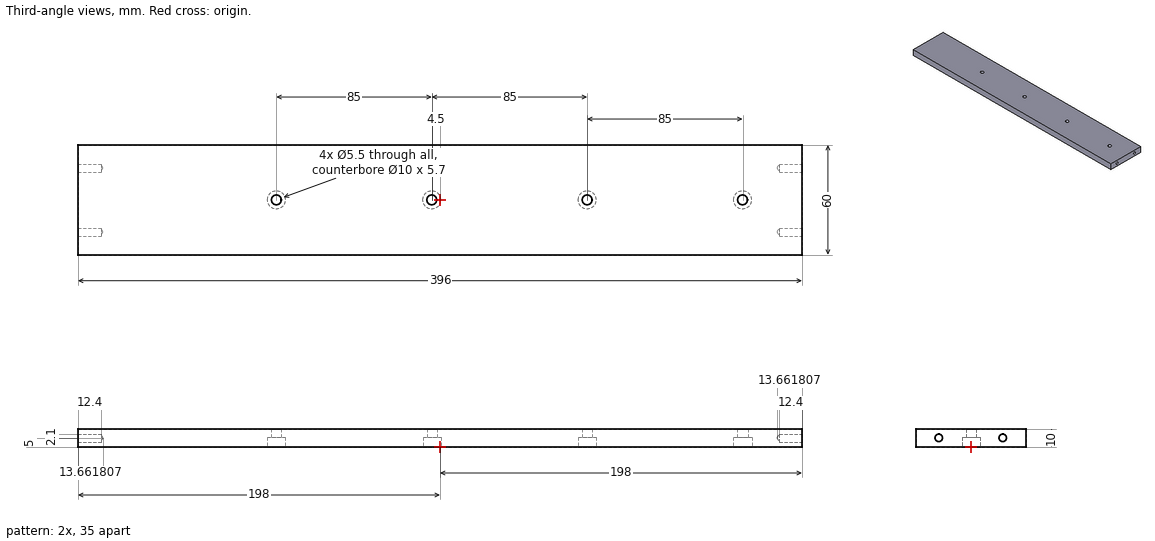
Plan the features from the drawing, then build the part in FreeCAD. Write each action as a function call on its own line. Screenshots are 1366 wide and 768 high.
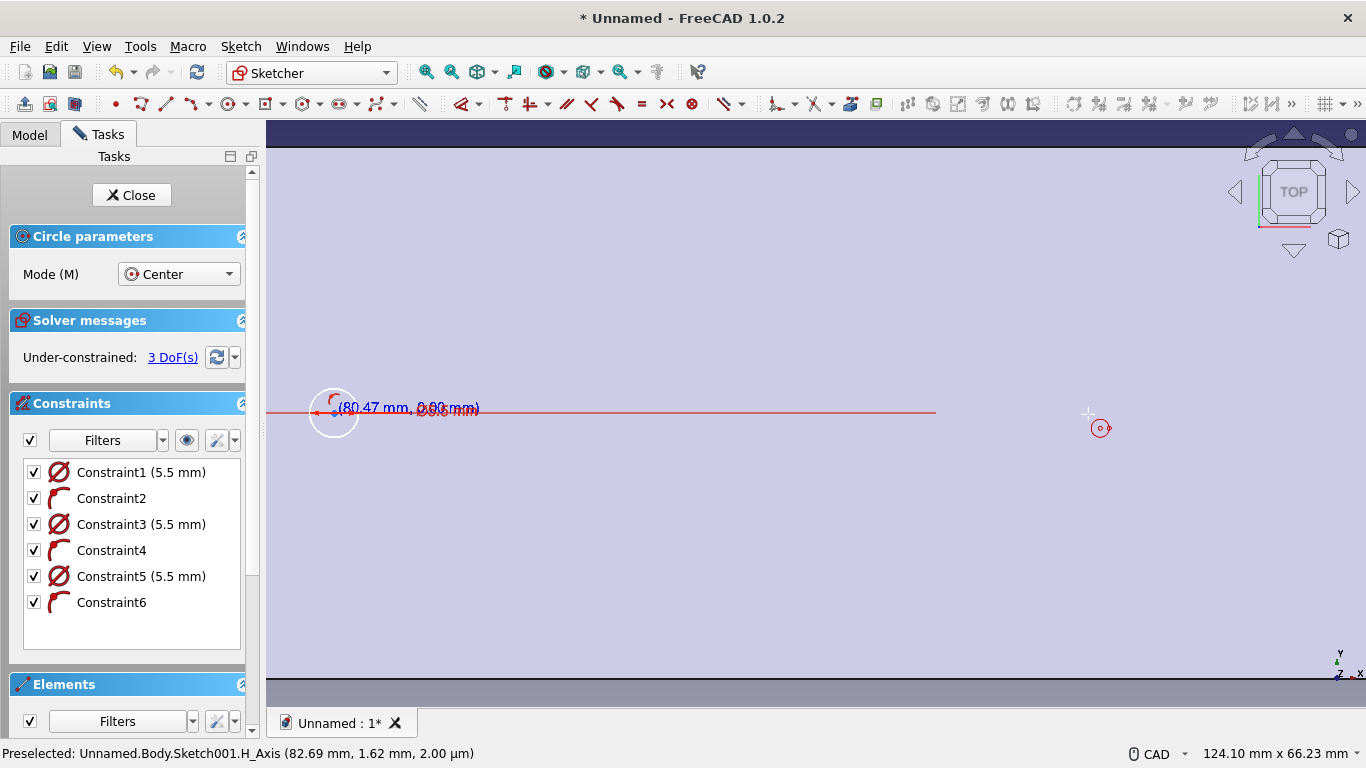
click(1088, 413)
move(1105, 396)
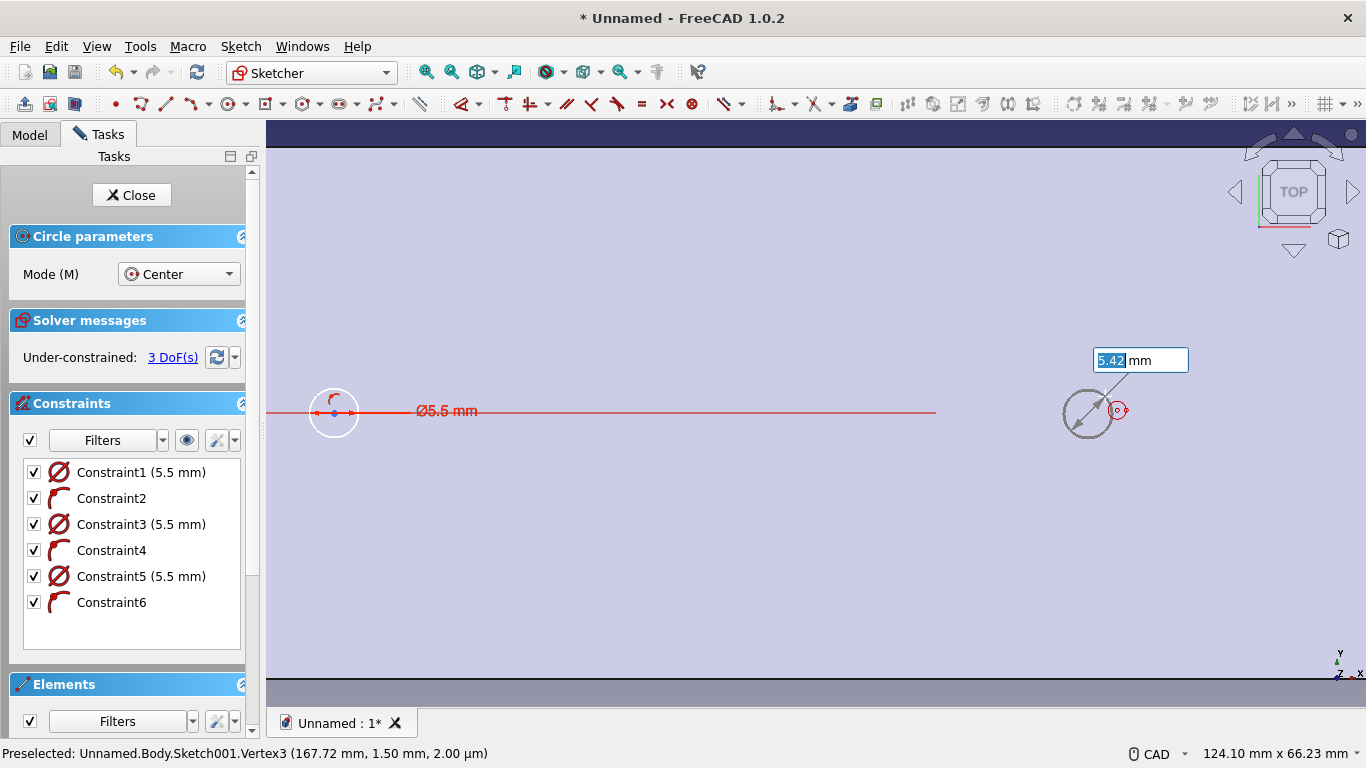
text(5.5)
key(Return)
key(Escape)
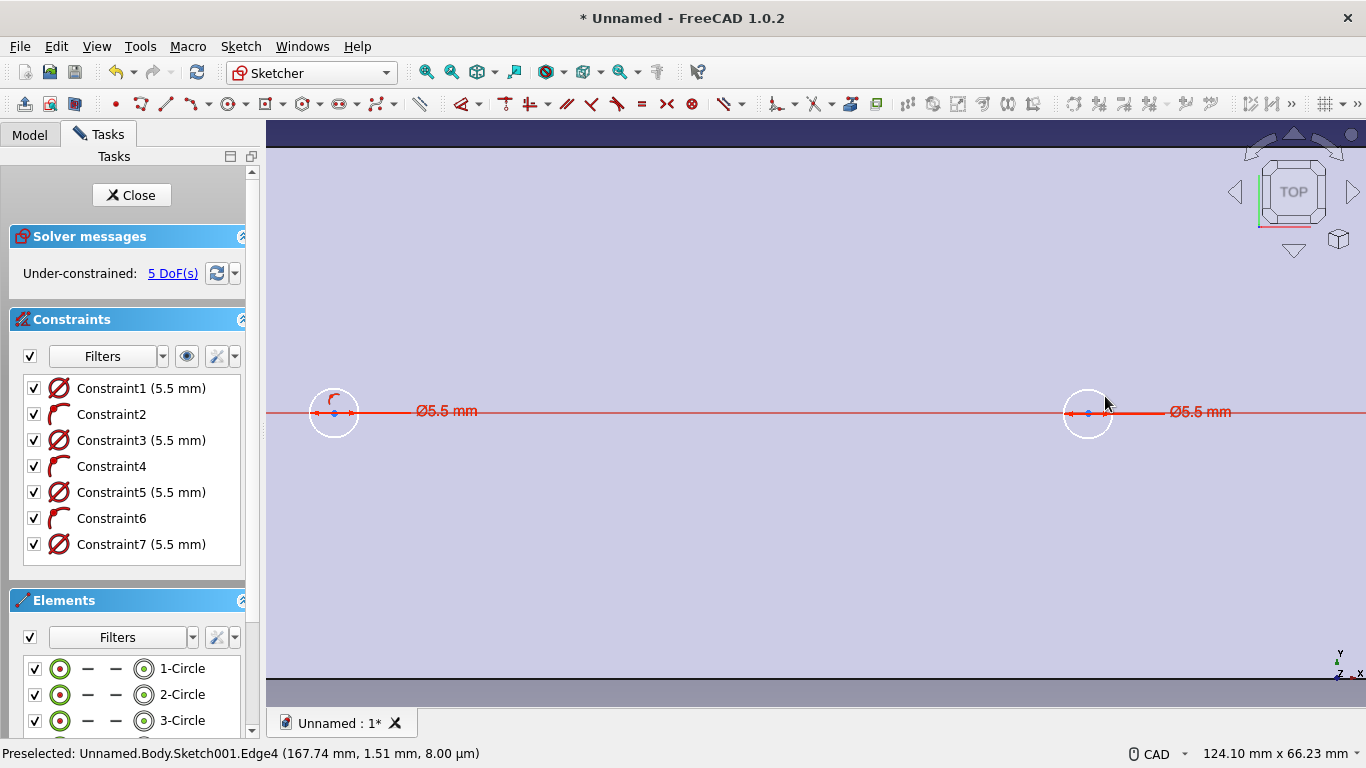
click(1088, 414)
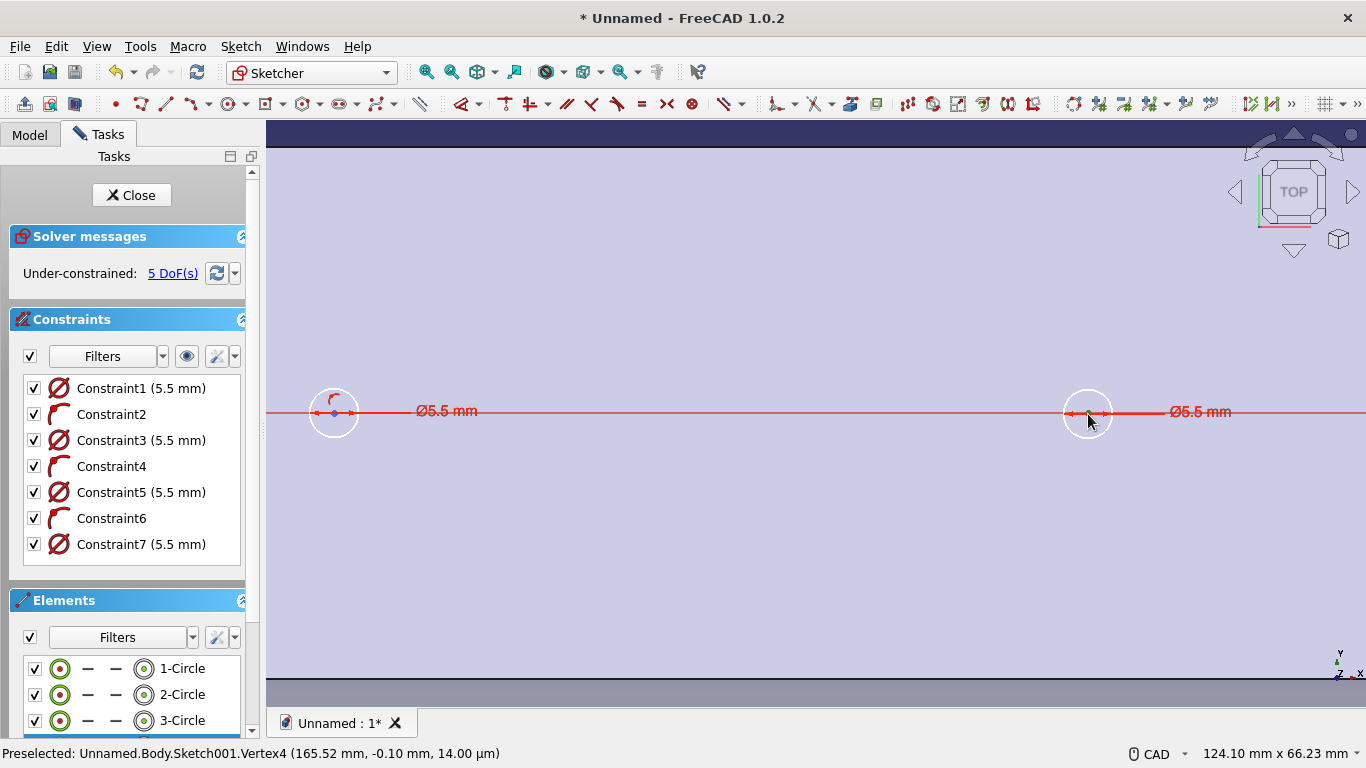
click(488, 413)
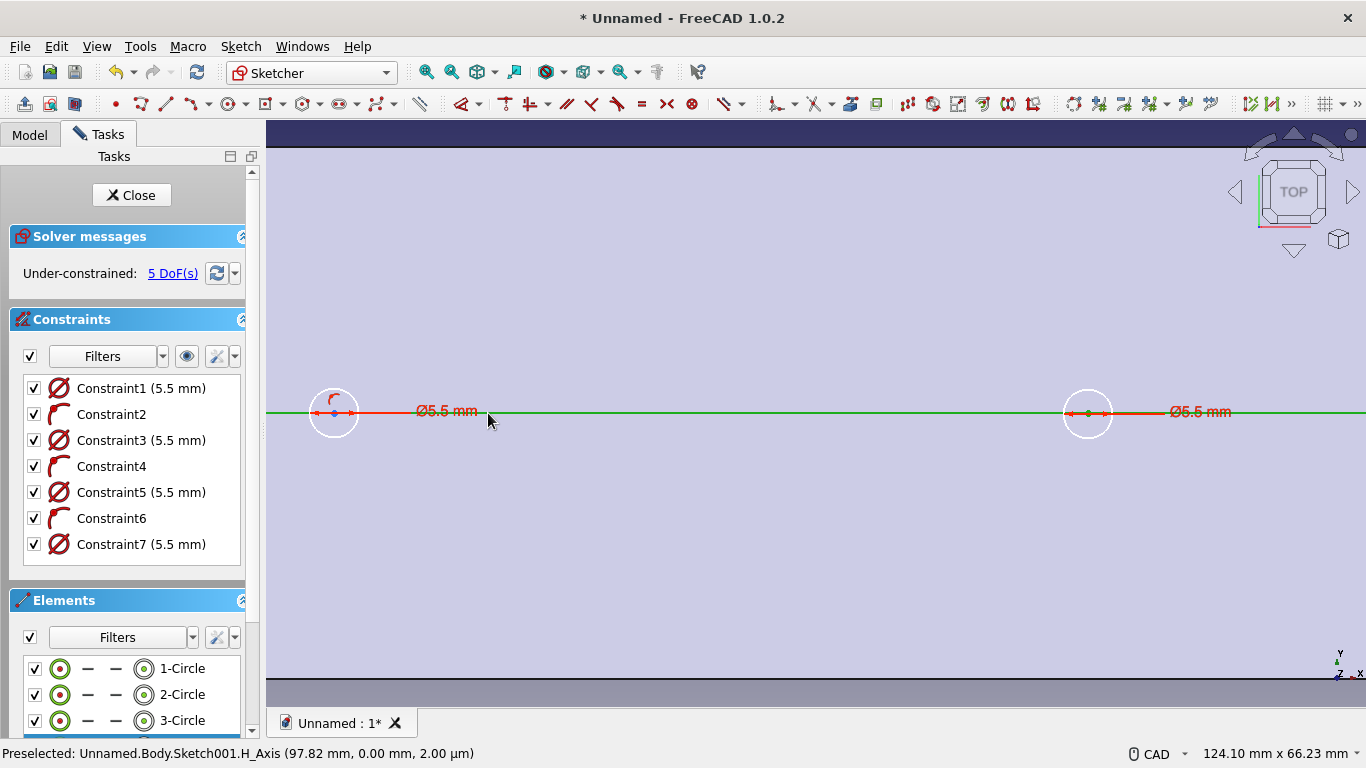
click(505, 104)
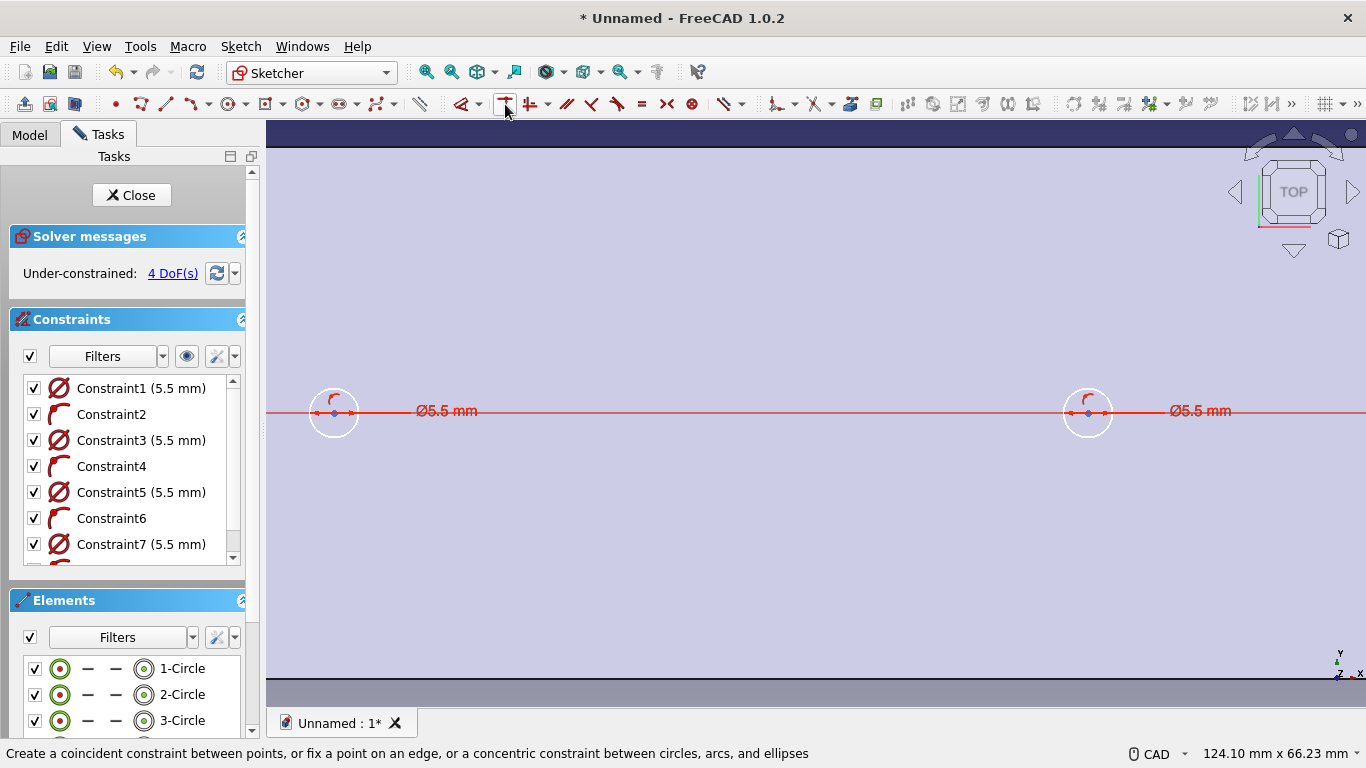
click(460, 104)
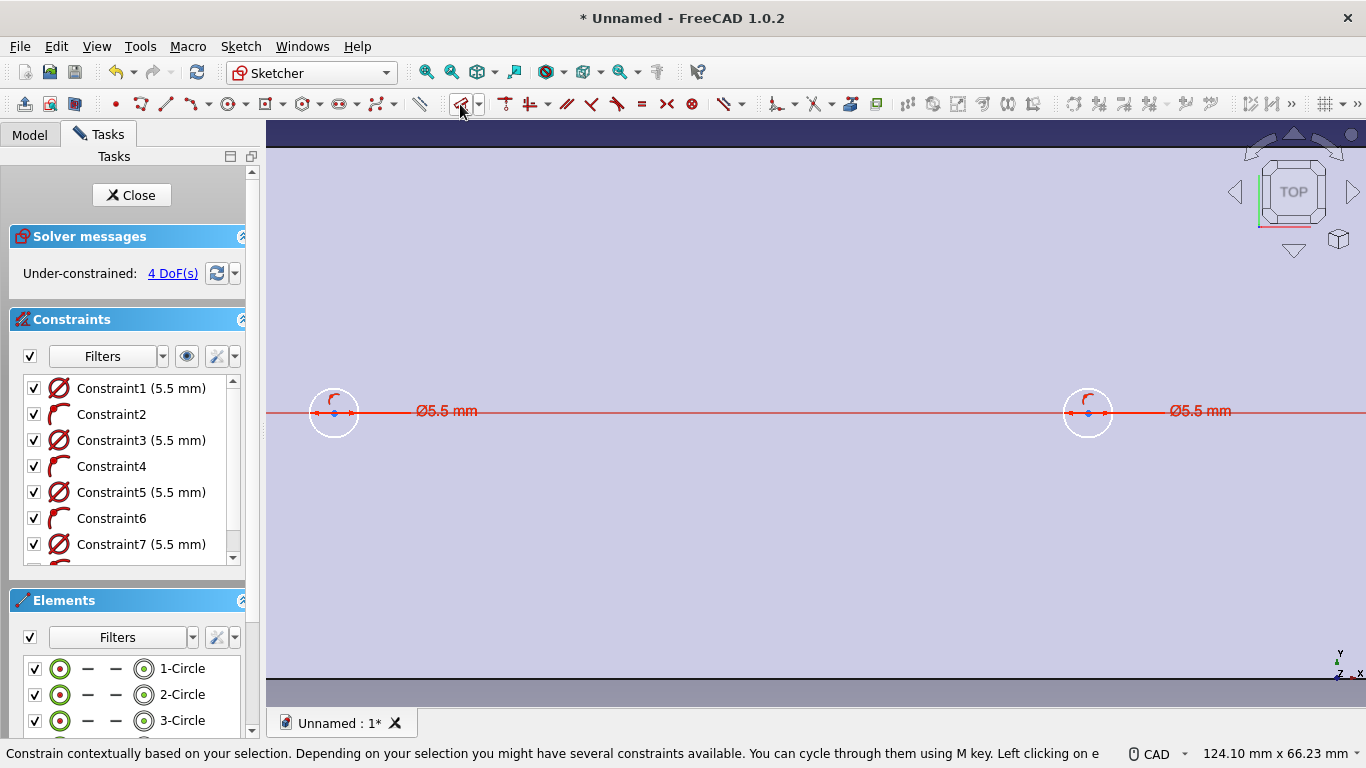
scroll(1088, 414, down, 6)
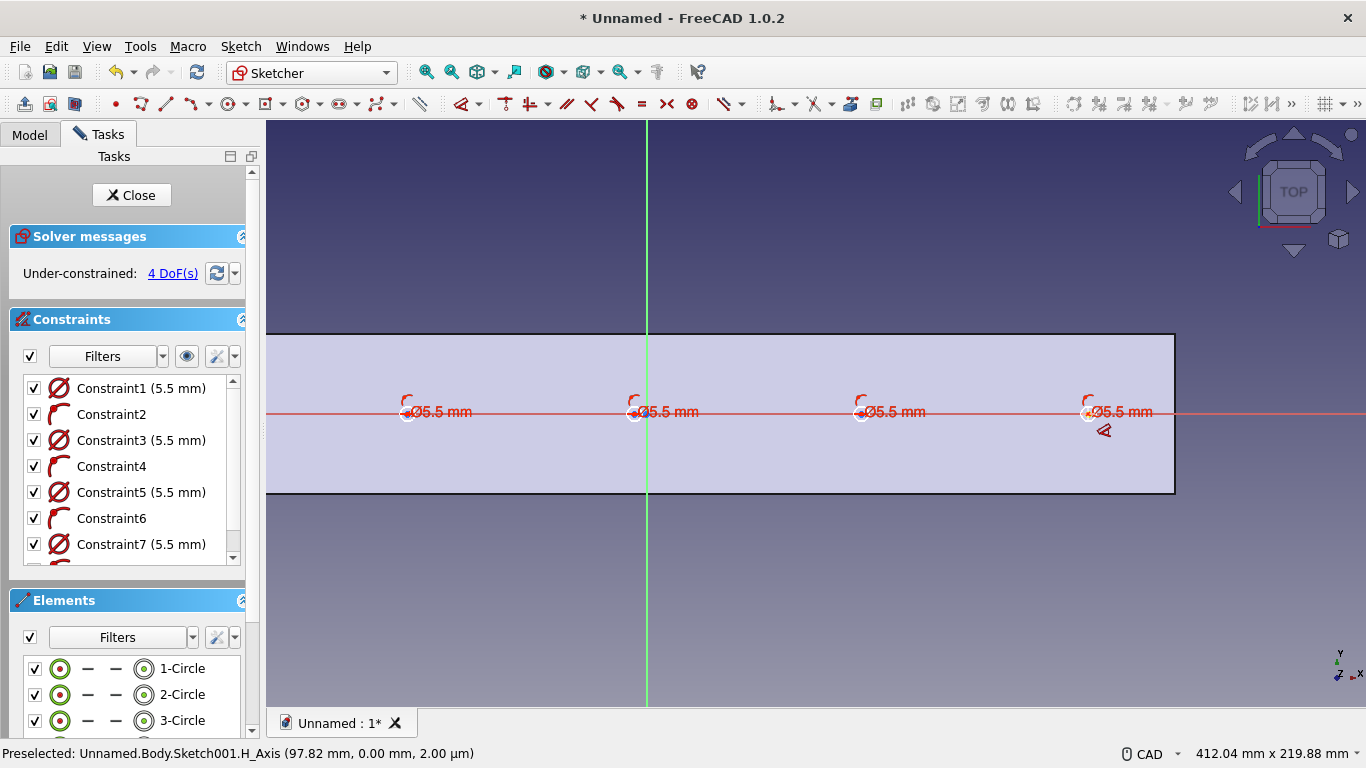
scroll(635, 414, up, 6)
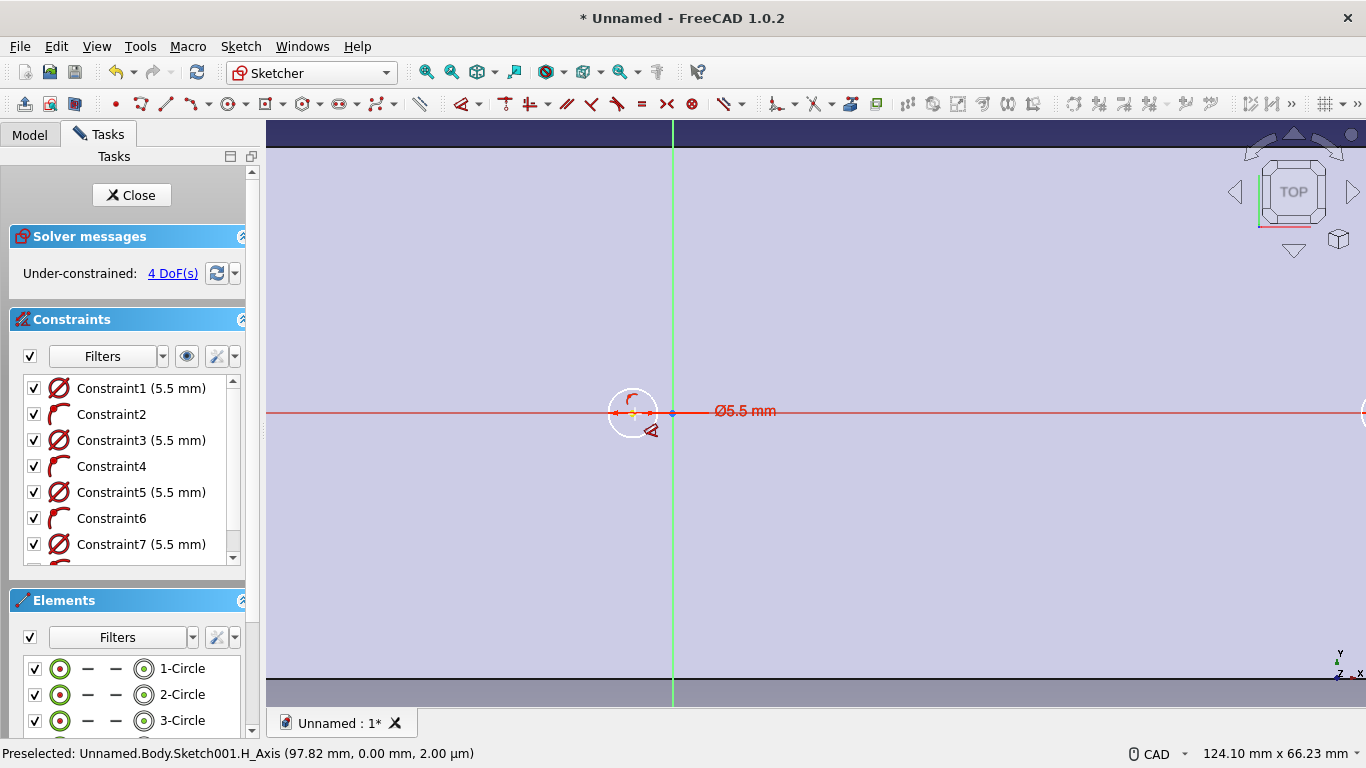
click(633, 413)
click(653, 447)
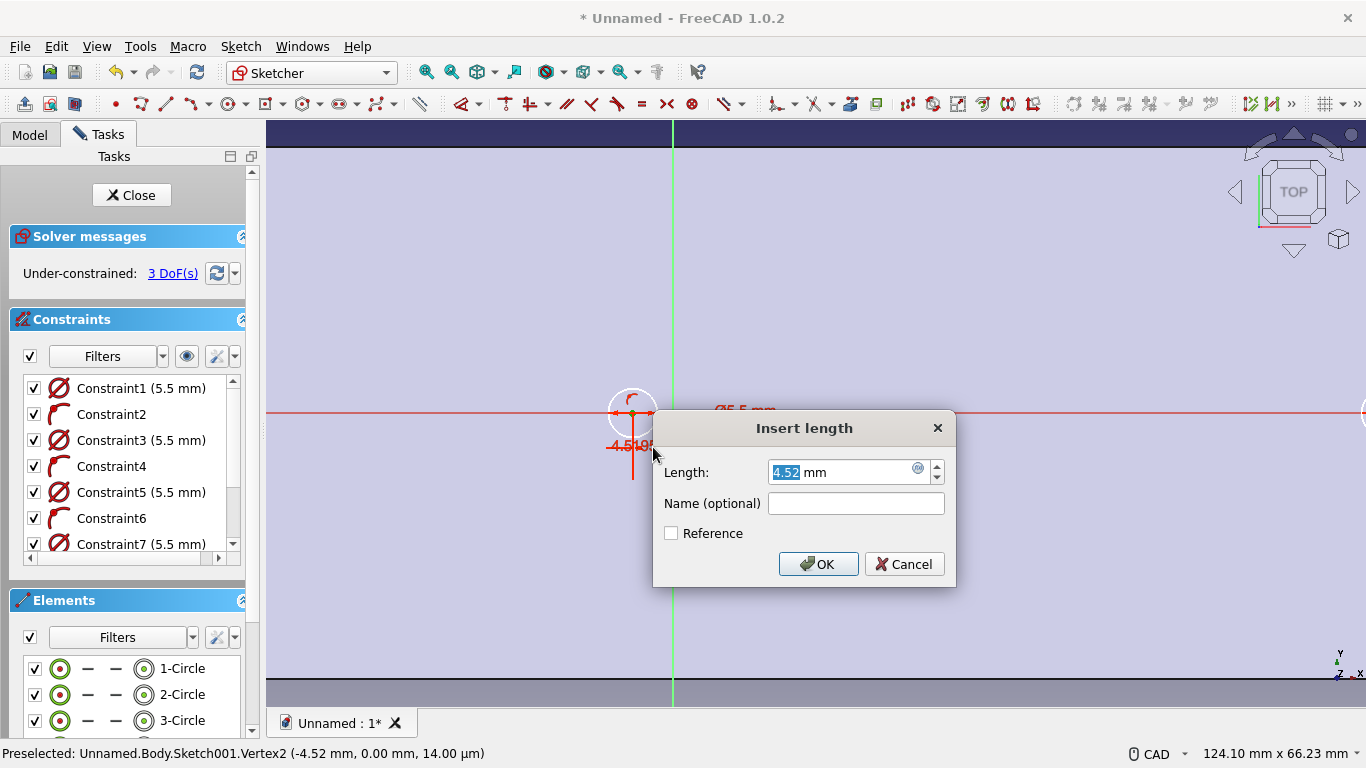
text(4.5)
key(Return)